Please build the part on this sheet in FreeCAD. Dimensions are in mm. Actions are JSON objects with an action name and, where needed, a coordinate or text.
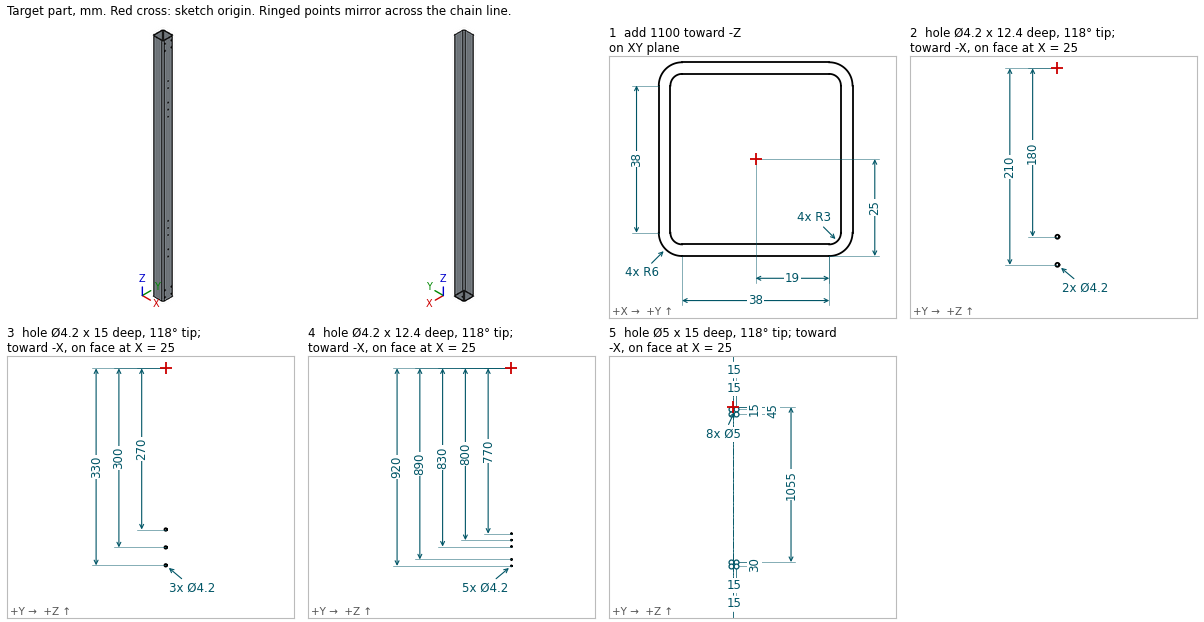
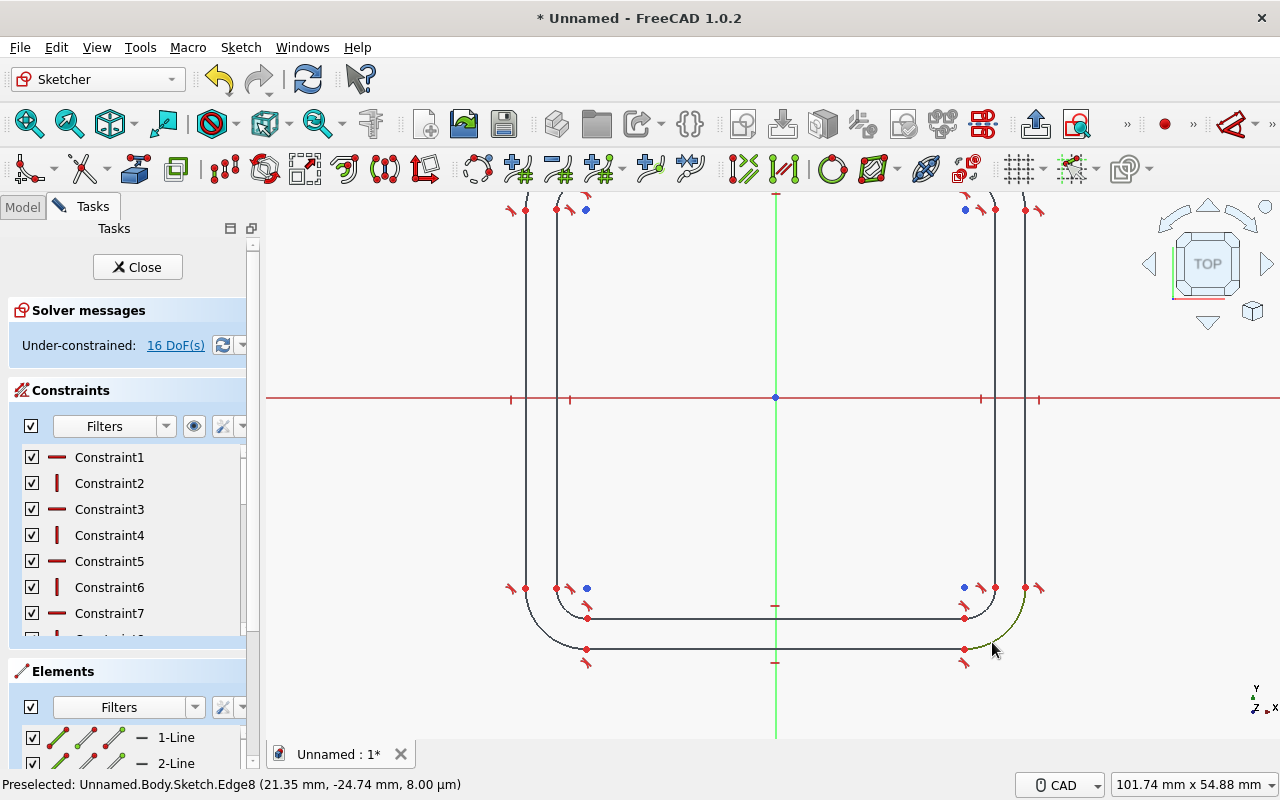
{"action": "left_click", "coordinate": [979, 615]}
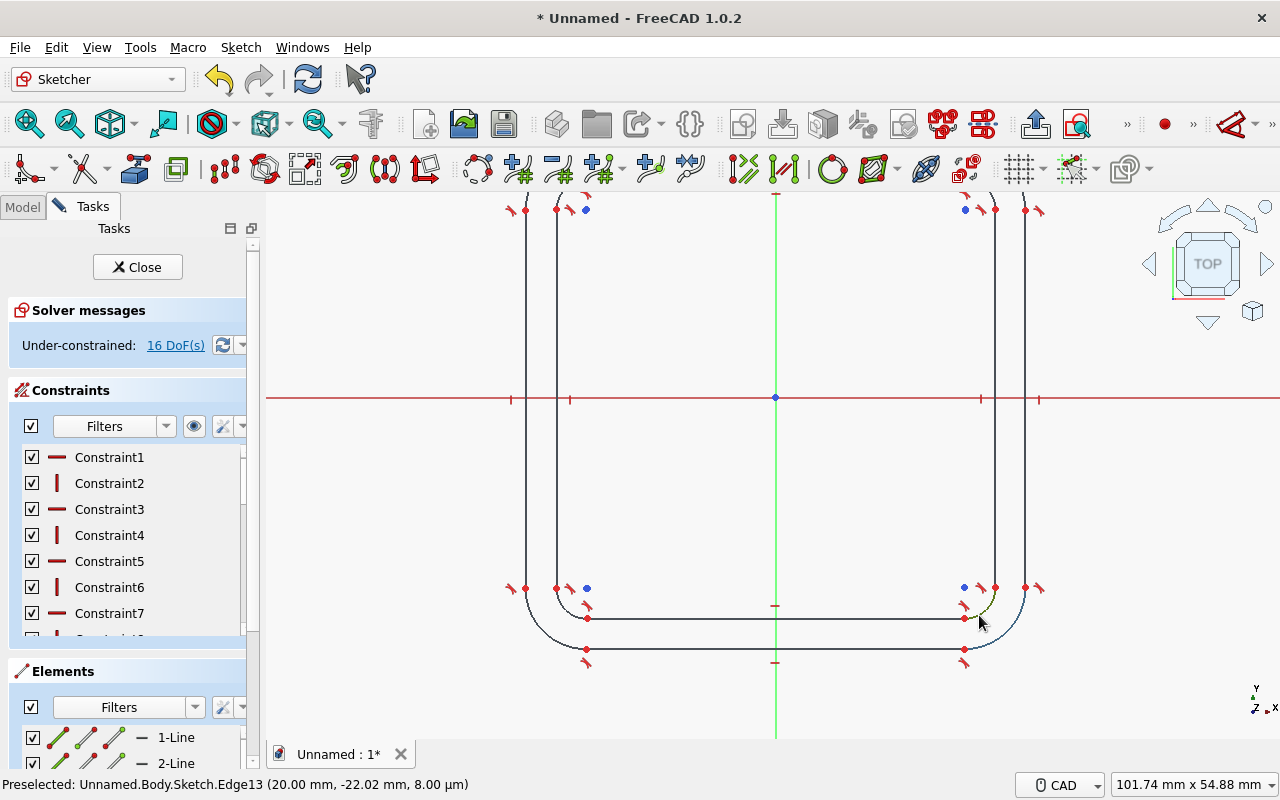
{"action": "key", "text": "c"}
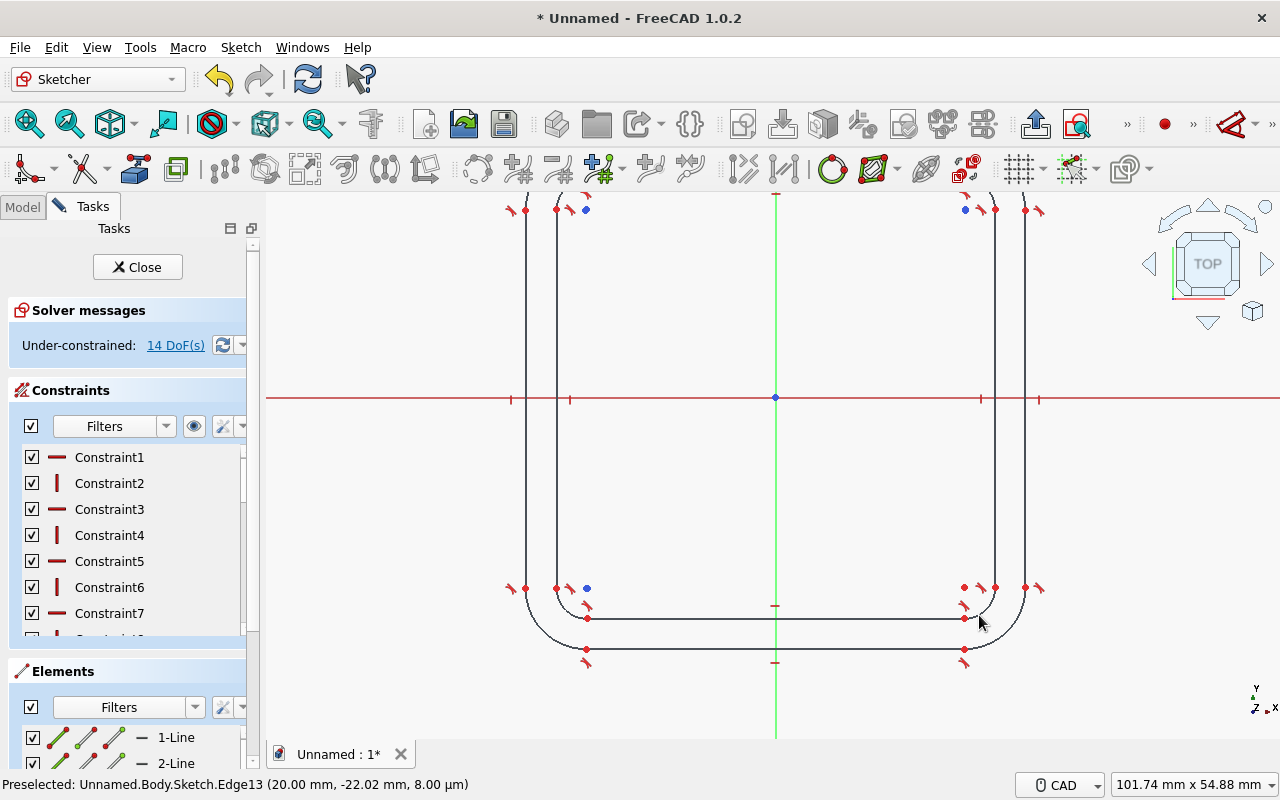
{"action": "scroll", "coordinate": [560, 604], "scroll_direction": "down", "scroll_amount": 2}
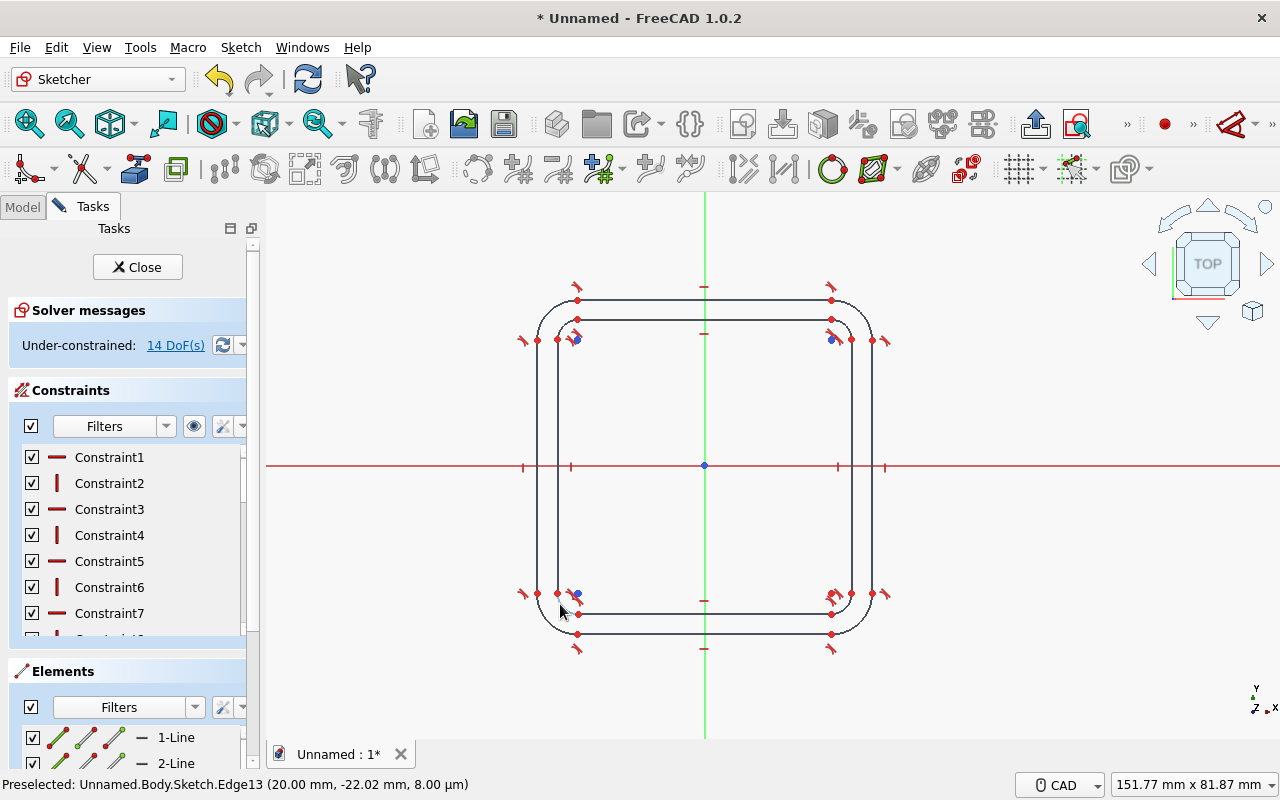
{"action": "left_click", "coordinate": [868, 322]}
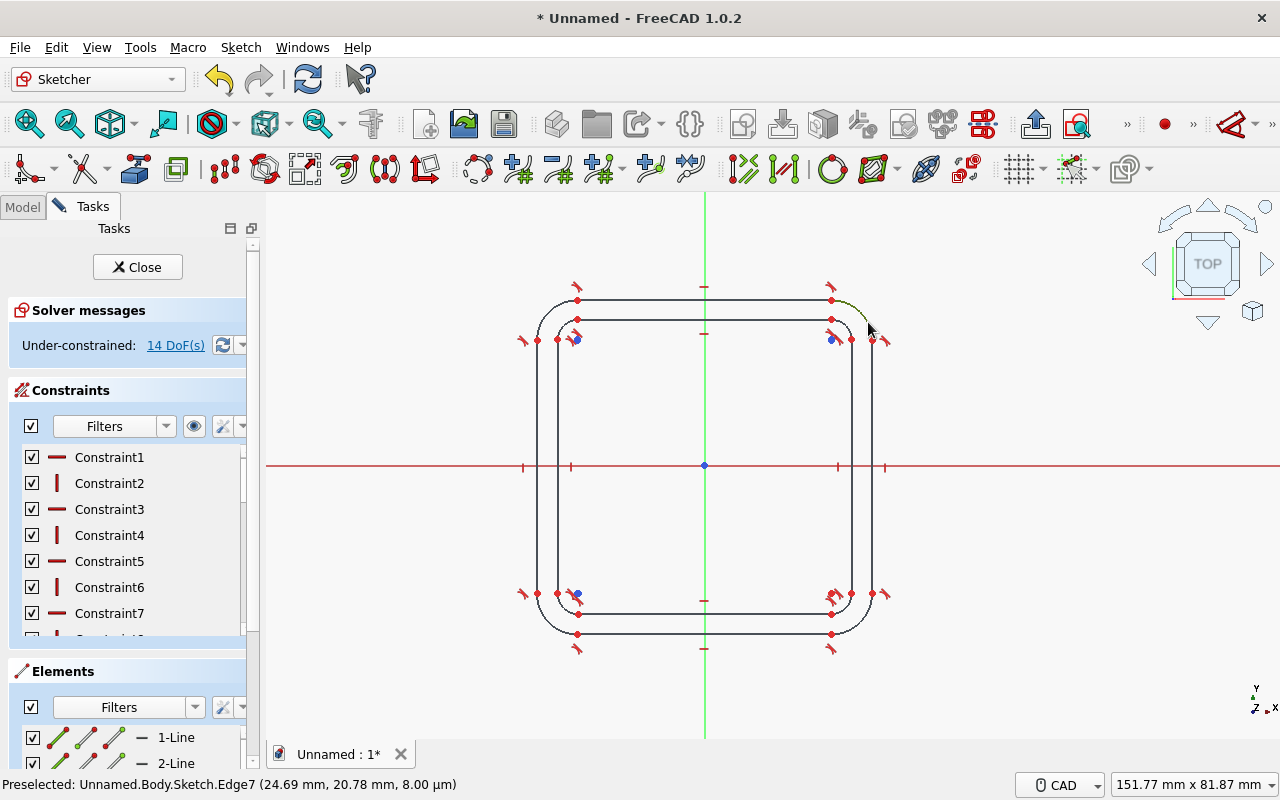
{"action": "scroll", "coordinate": [850, 331], "scroll_direction": "up", "scroll_amount": 3}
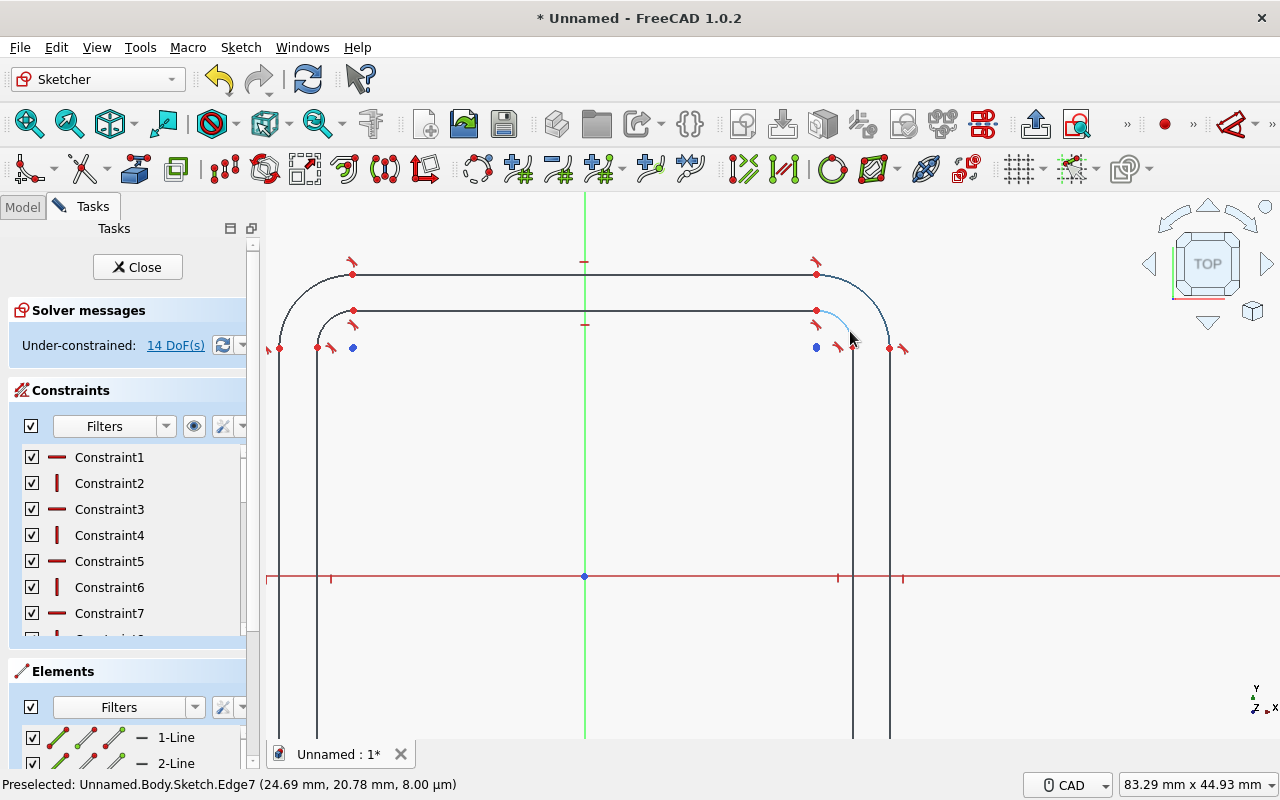
{"action": "left_click", "coordinate": [849, 330]}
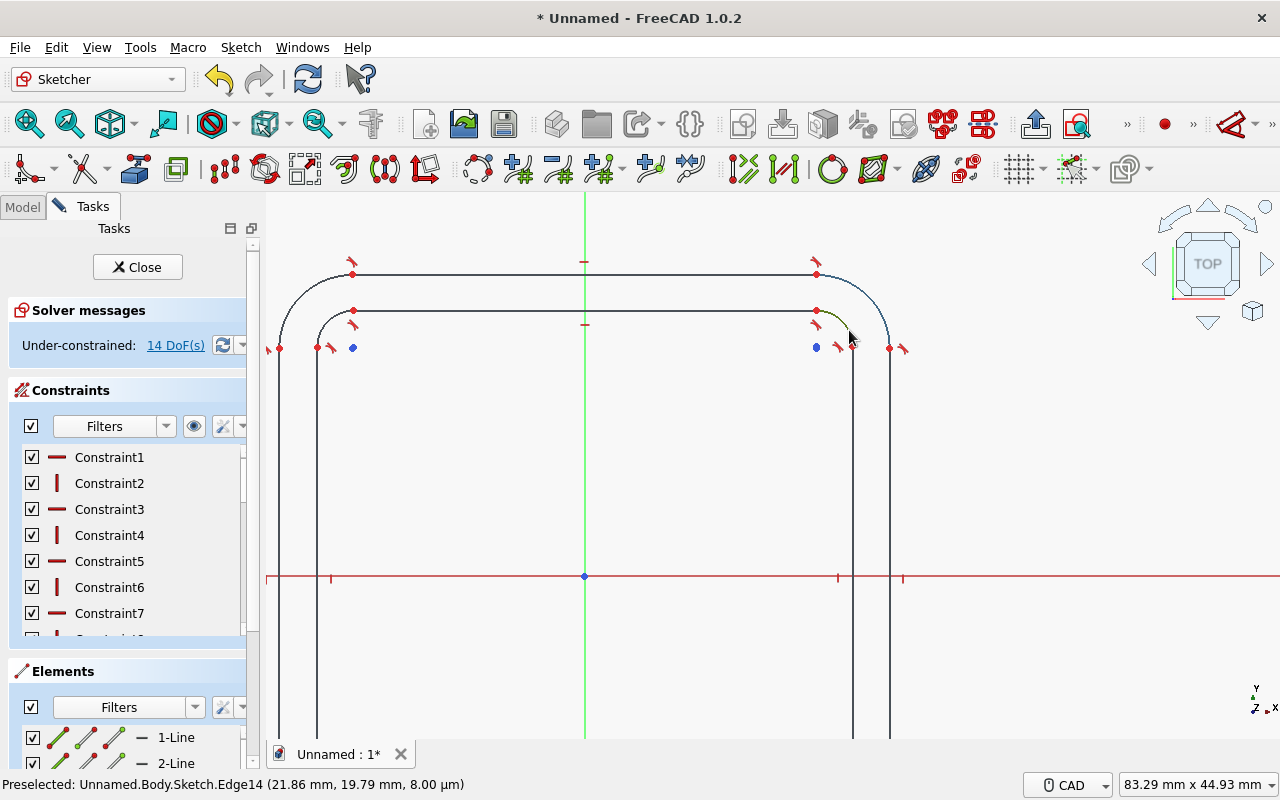
{"action": "key", "text": "c"}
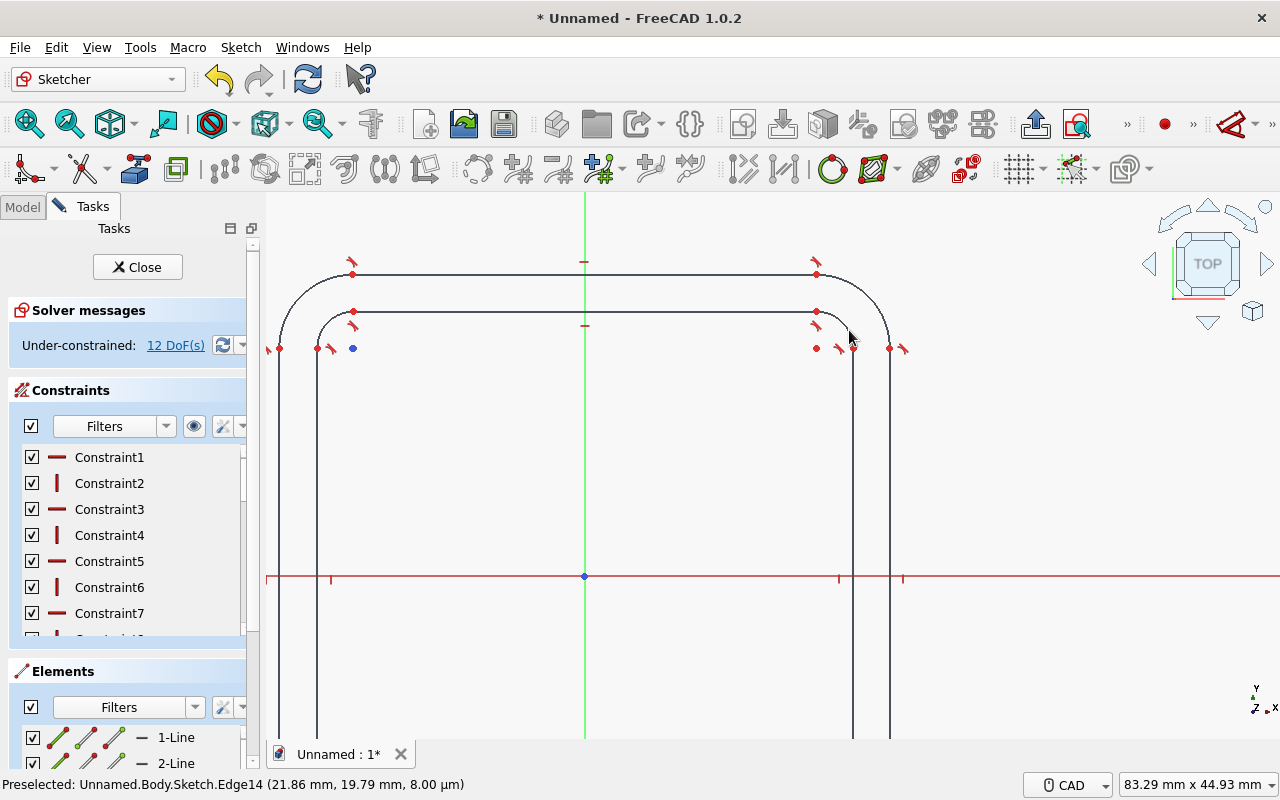
{"action": "left_click", "coordinate": [319, 283]}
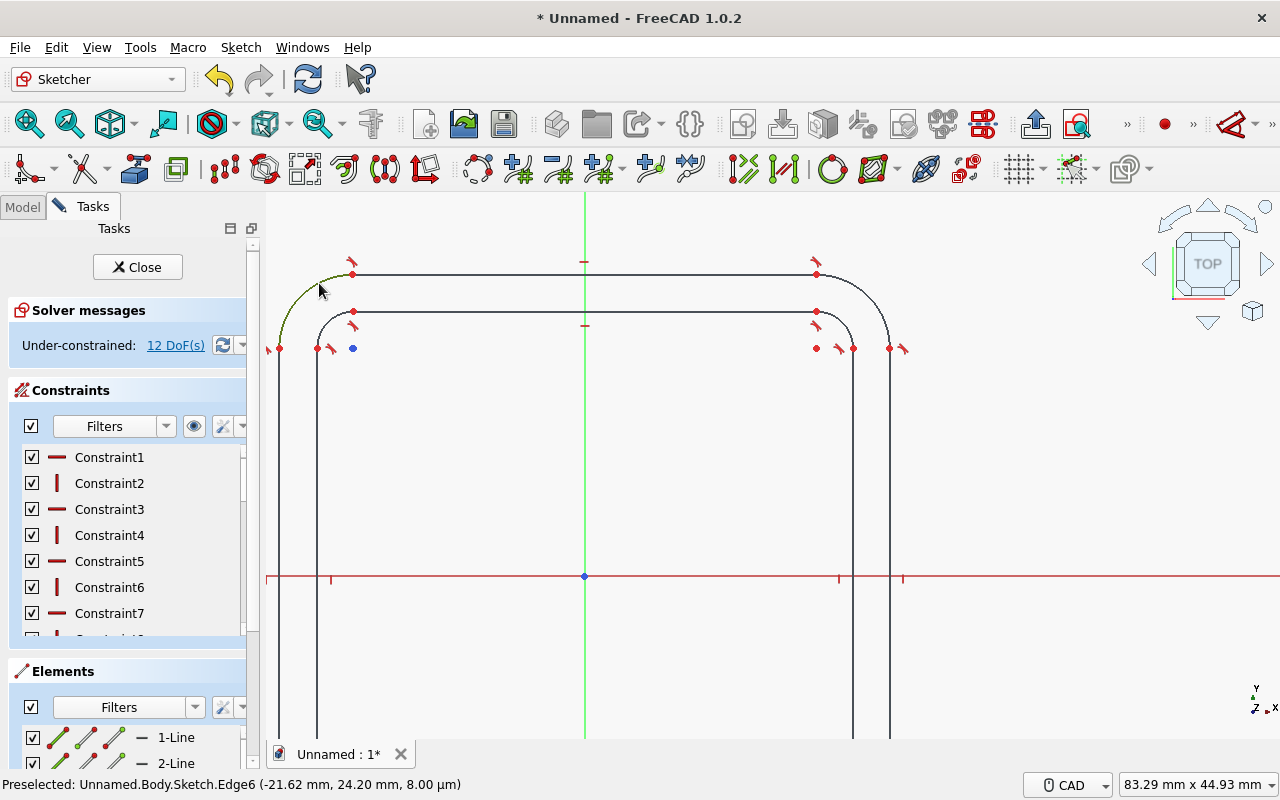
{"action": "left_click", "coordinate": [337, 316]}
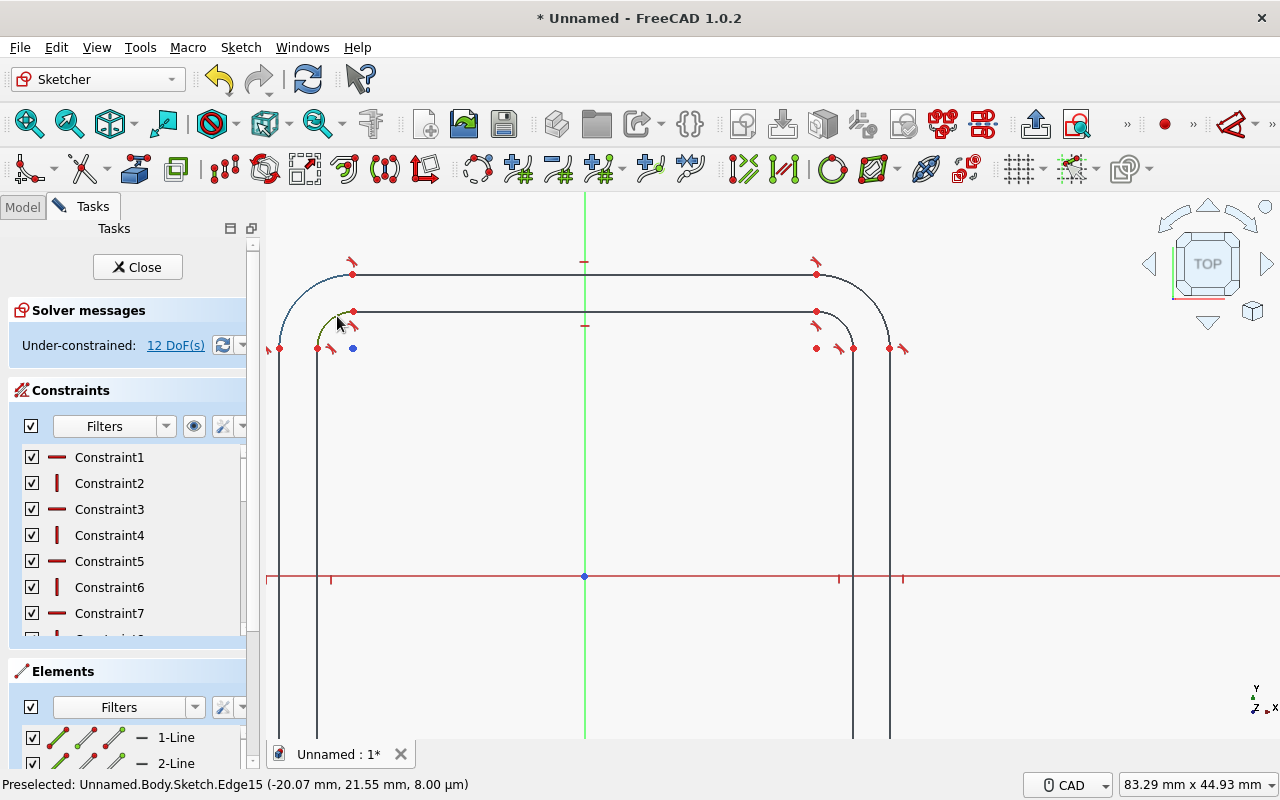
{"action": "key", "text": "c"}